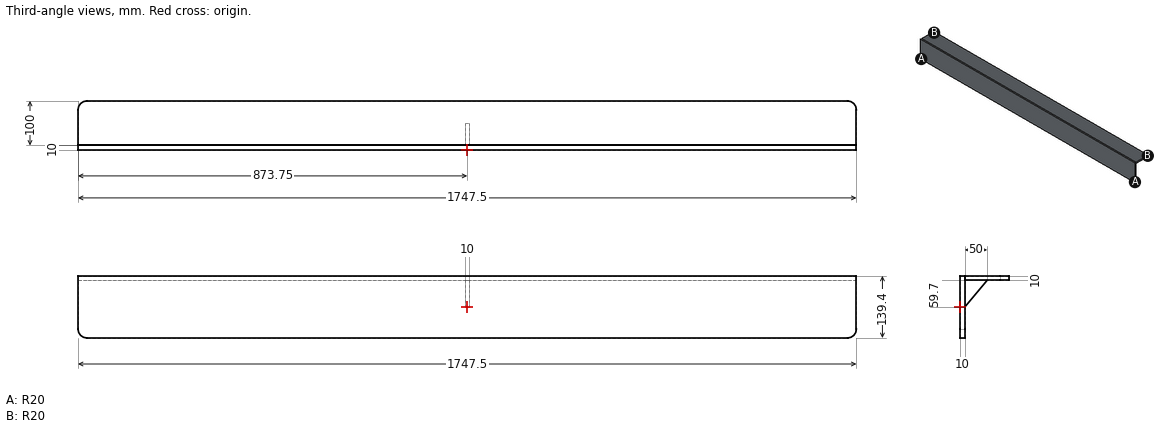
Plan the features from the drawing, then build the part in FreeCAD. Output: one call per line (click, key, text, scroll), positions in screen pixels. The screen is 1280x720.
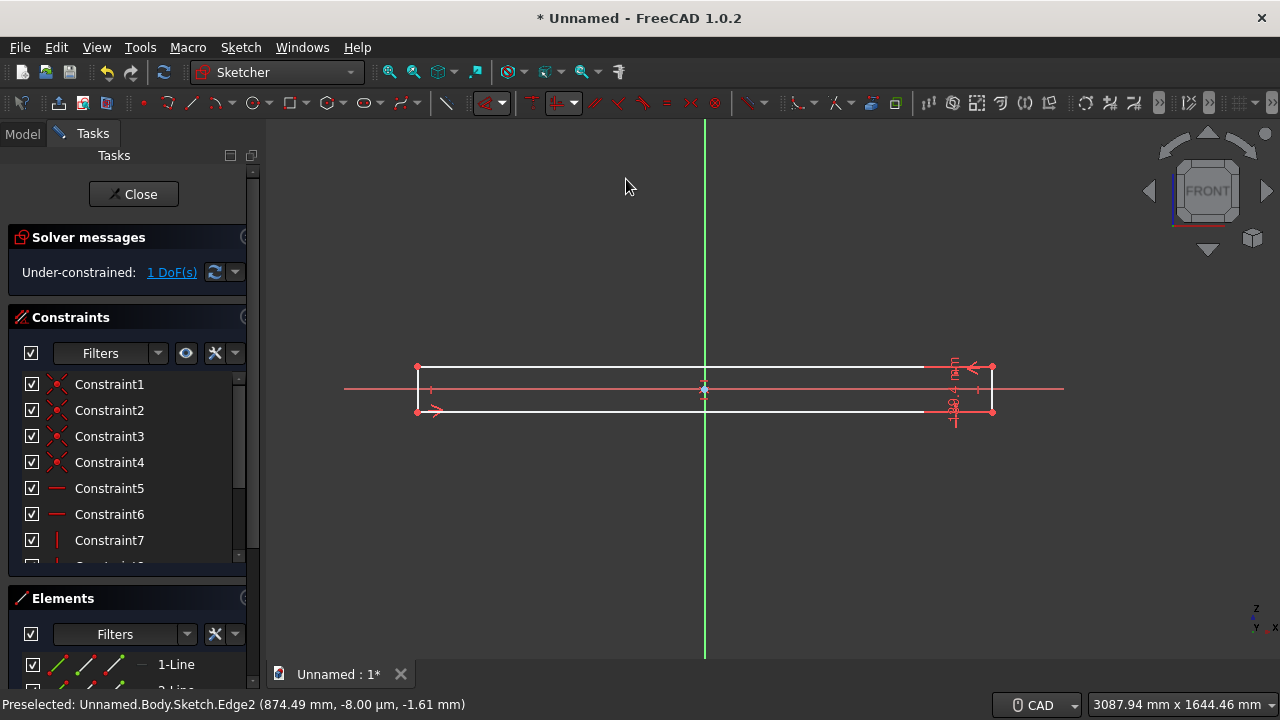
click(590, 412)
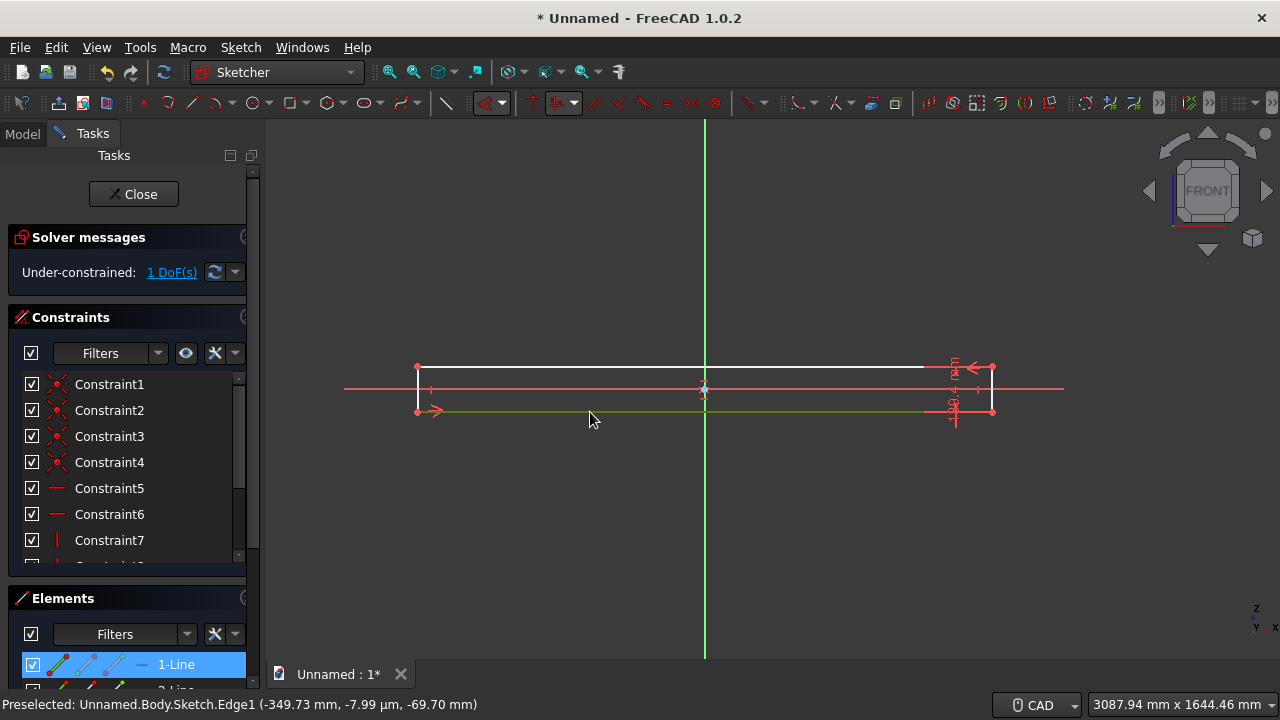
key(l)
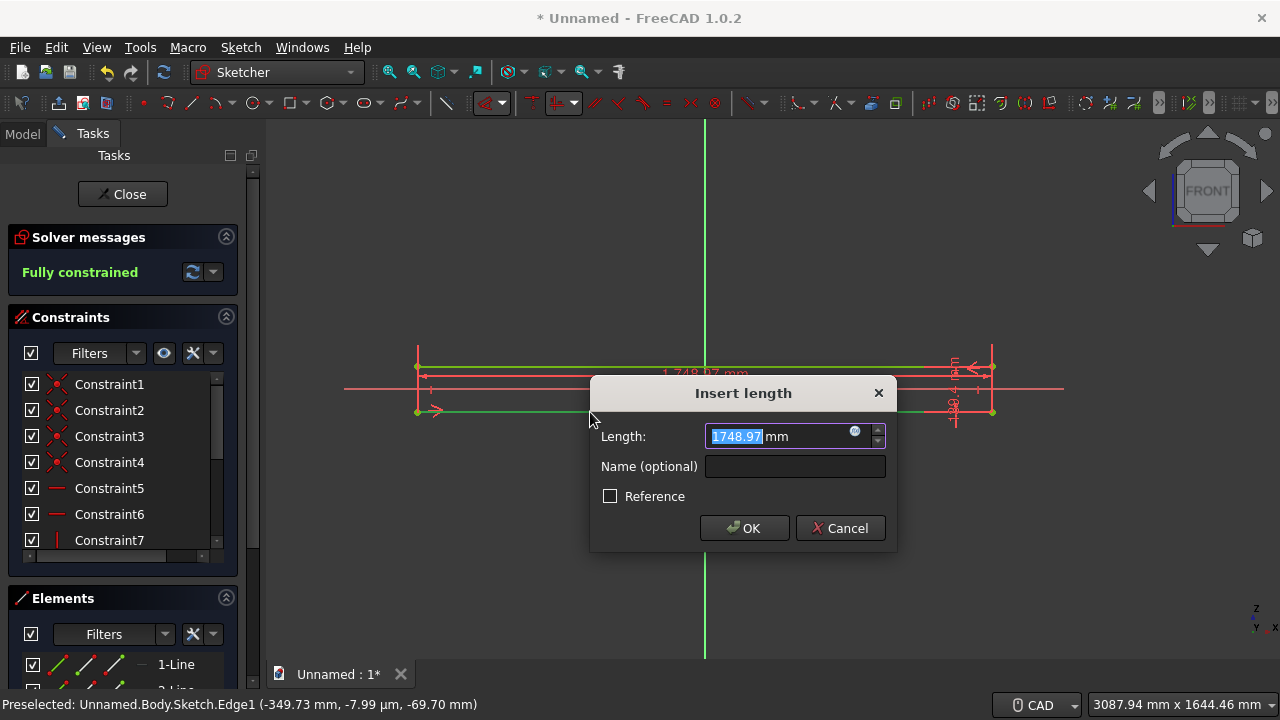
text(1747.5)
key(Return)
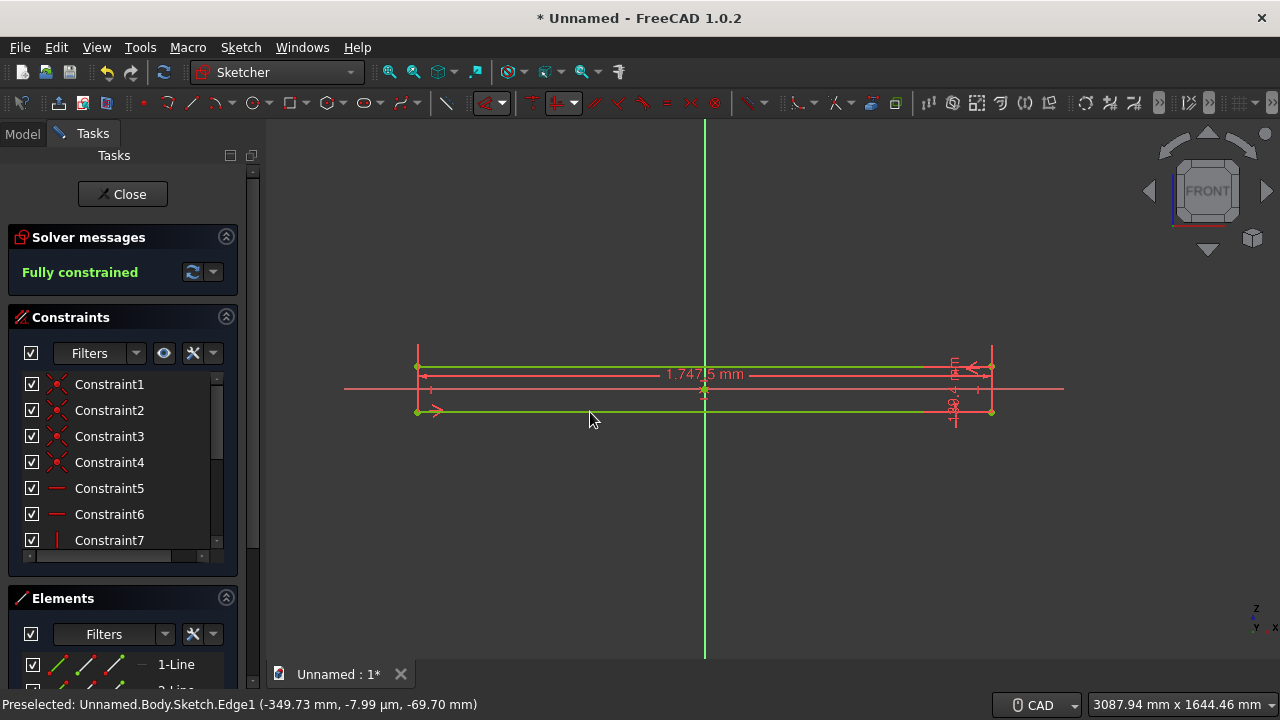
click(123, 194)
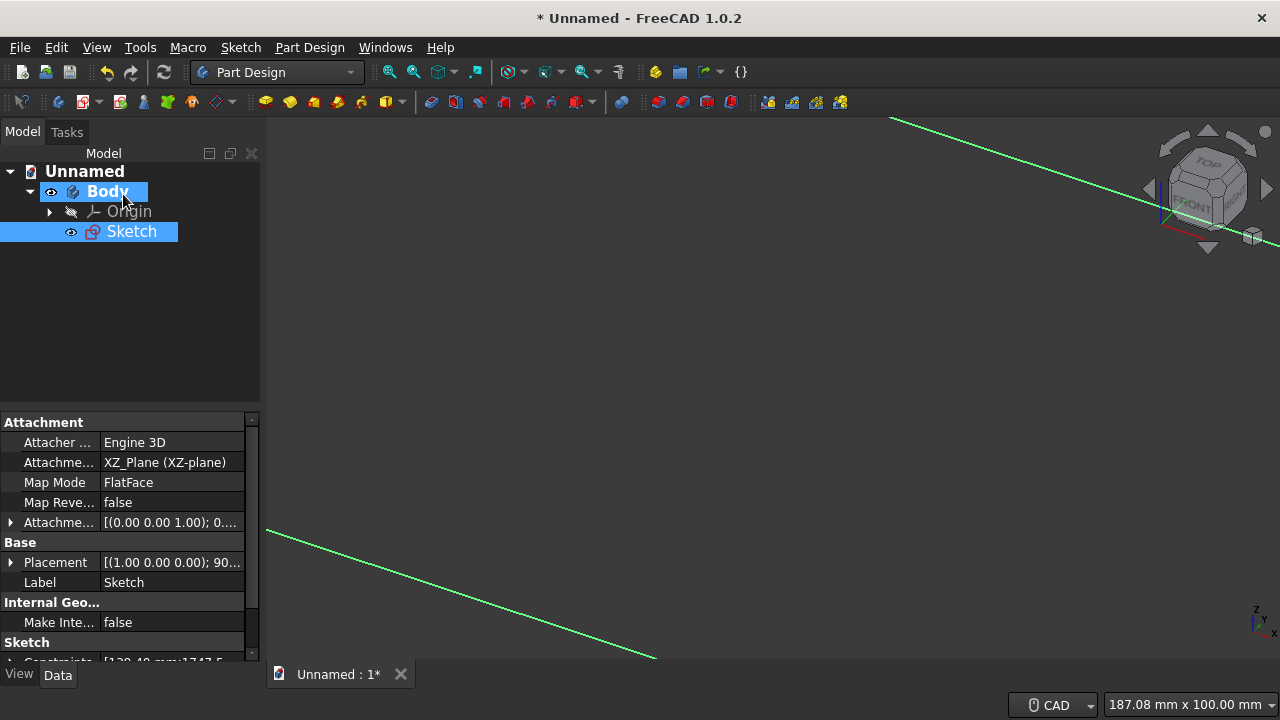
click(266, 102)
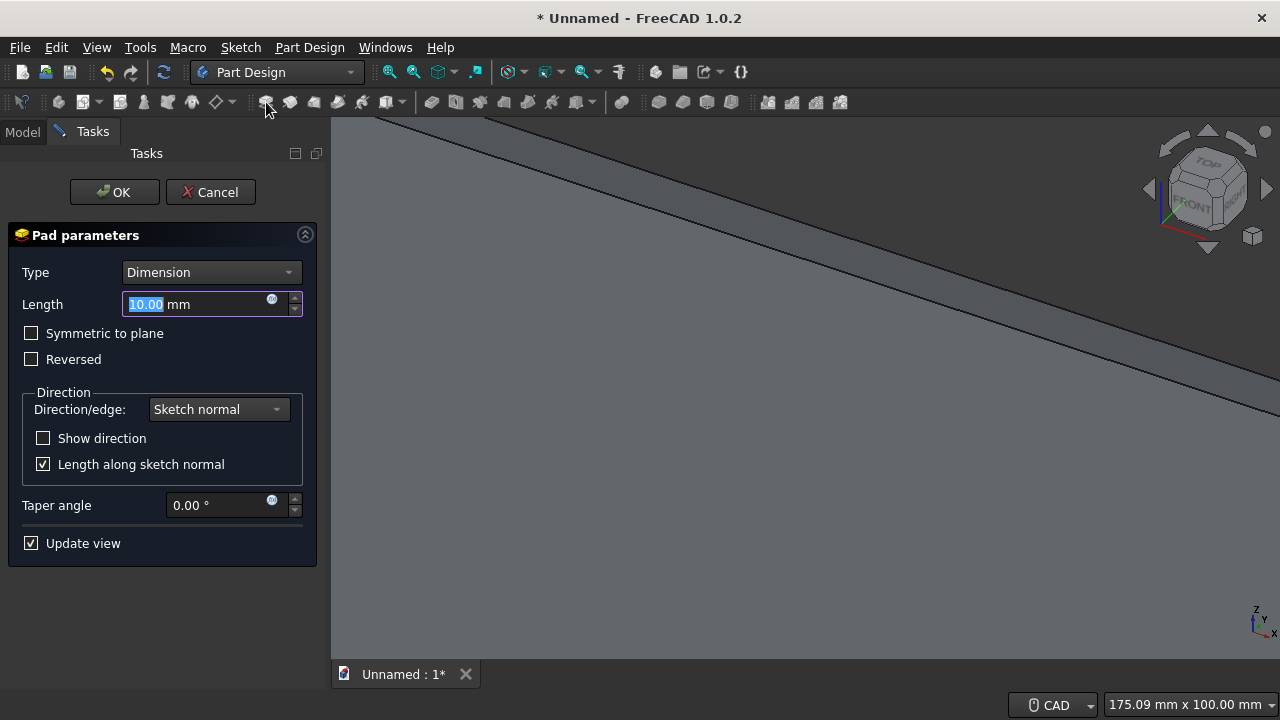
text(10)
key(Tab)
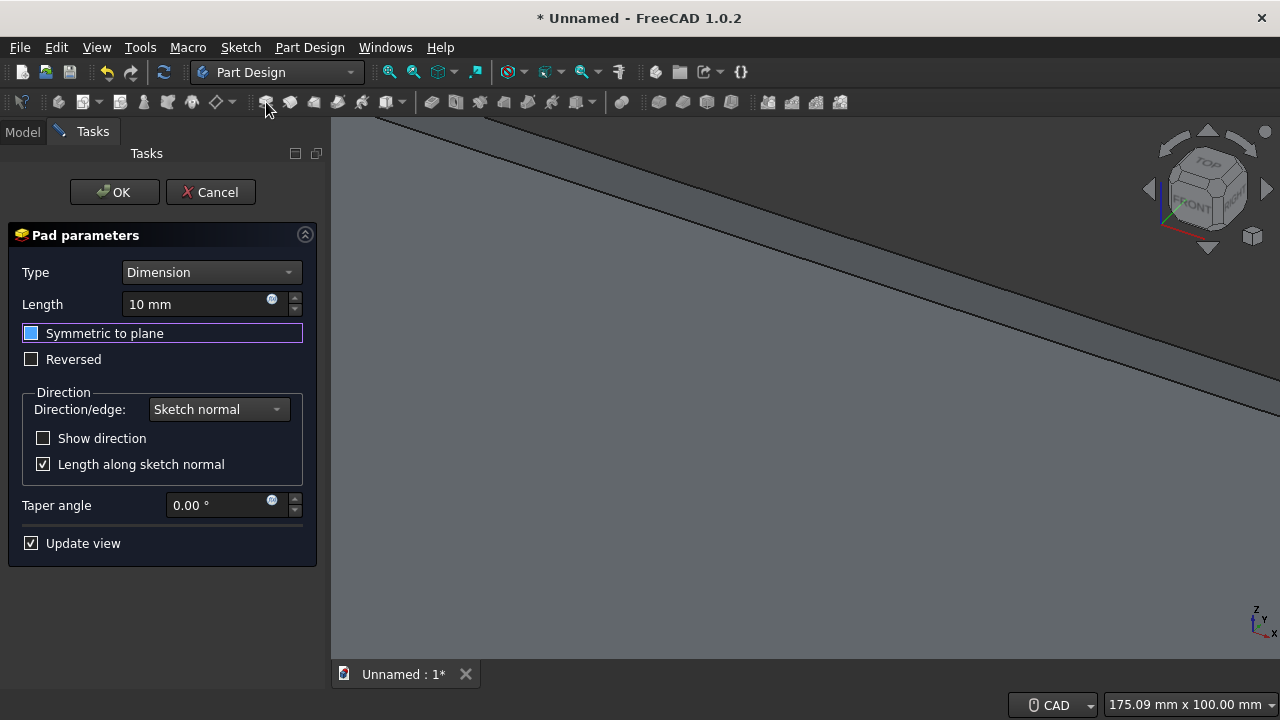
click(30, 359)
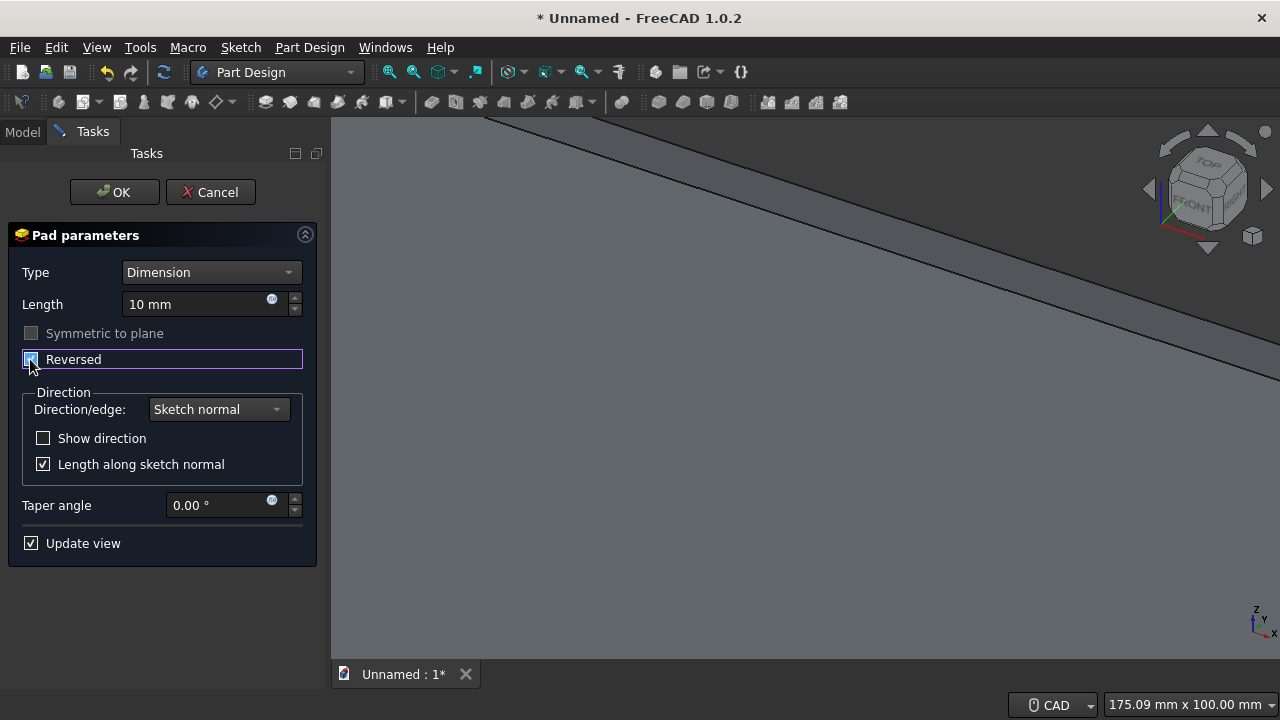
click(115, 192)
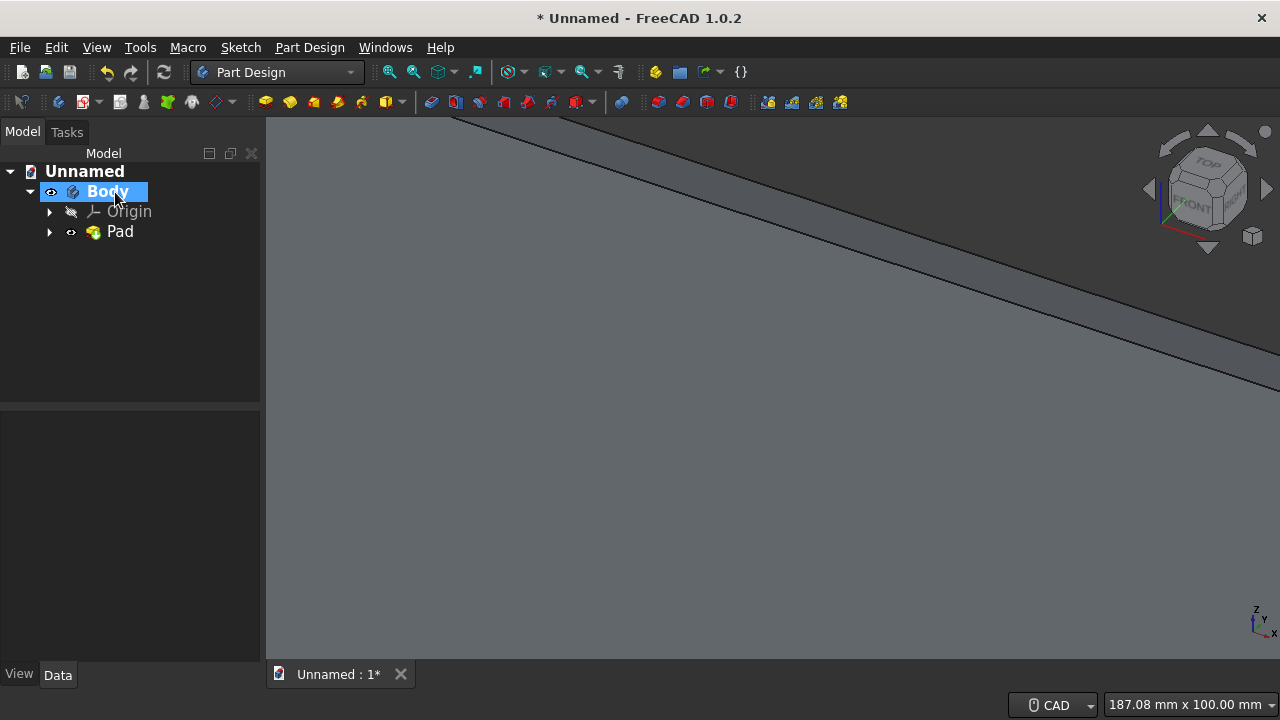
click(390, 72)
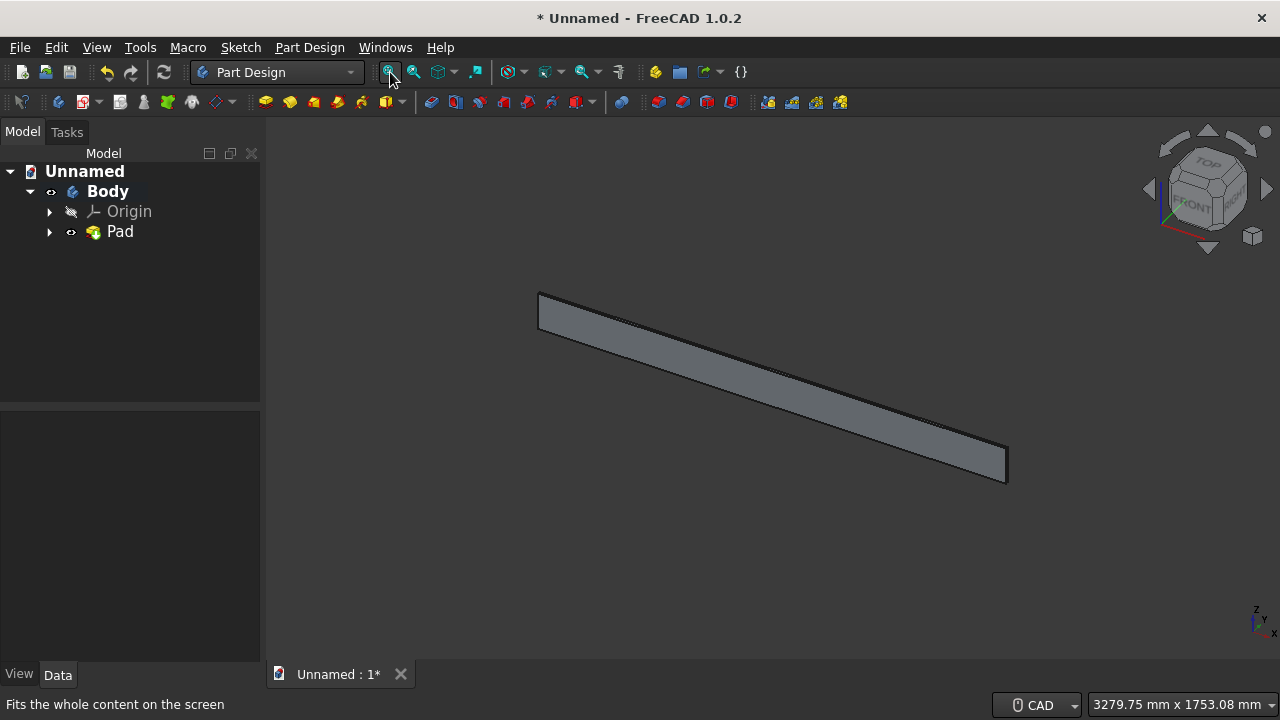
scroll(539, 327, up, 13)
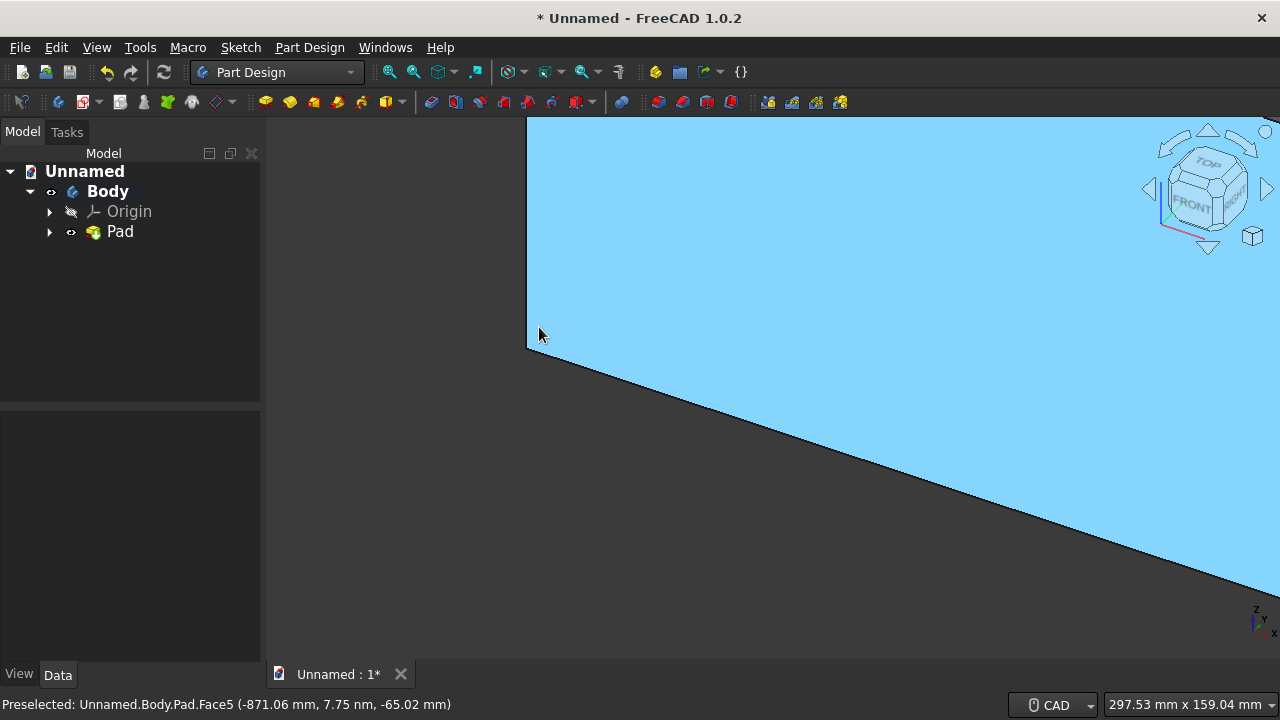
click(390, 72)